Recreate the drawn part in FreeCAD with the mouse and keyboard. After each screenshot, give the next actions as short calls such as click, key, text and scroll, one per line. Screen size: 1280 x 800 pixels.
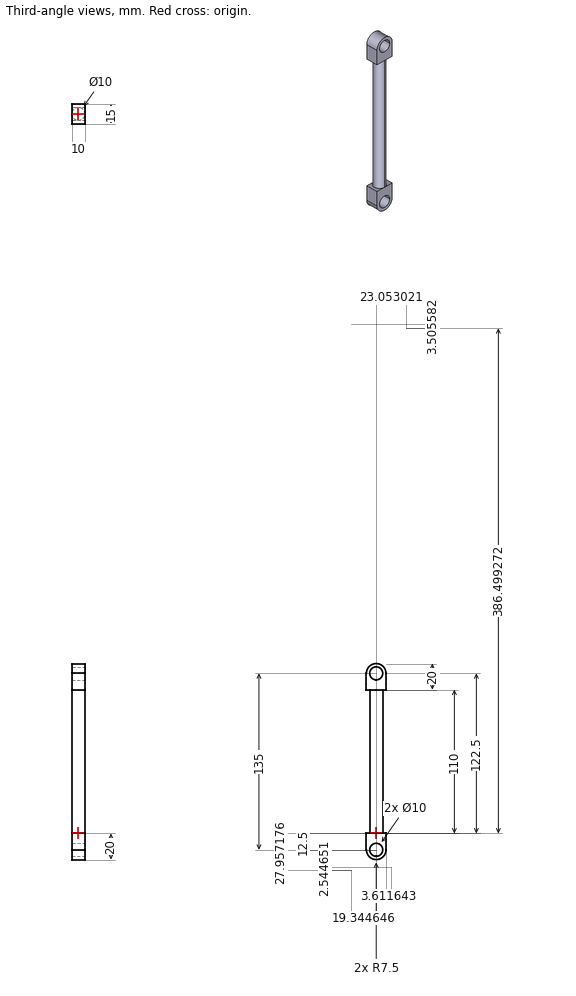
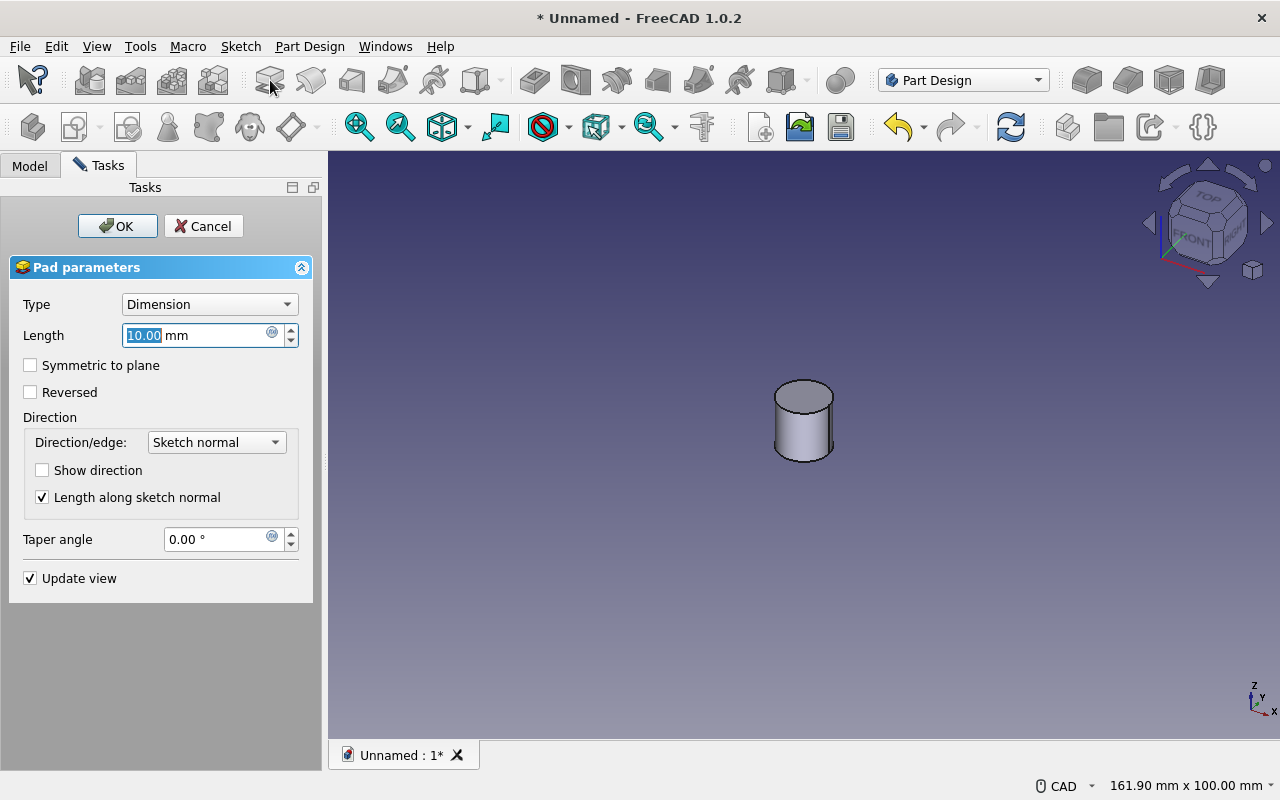
text(110)
key(Tab)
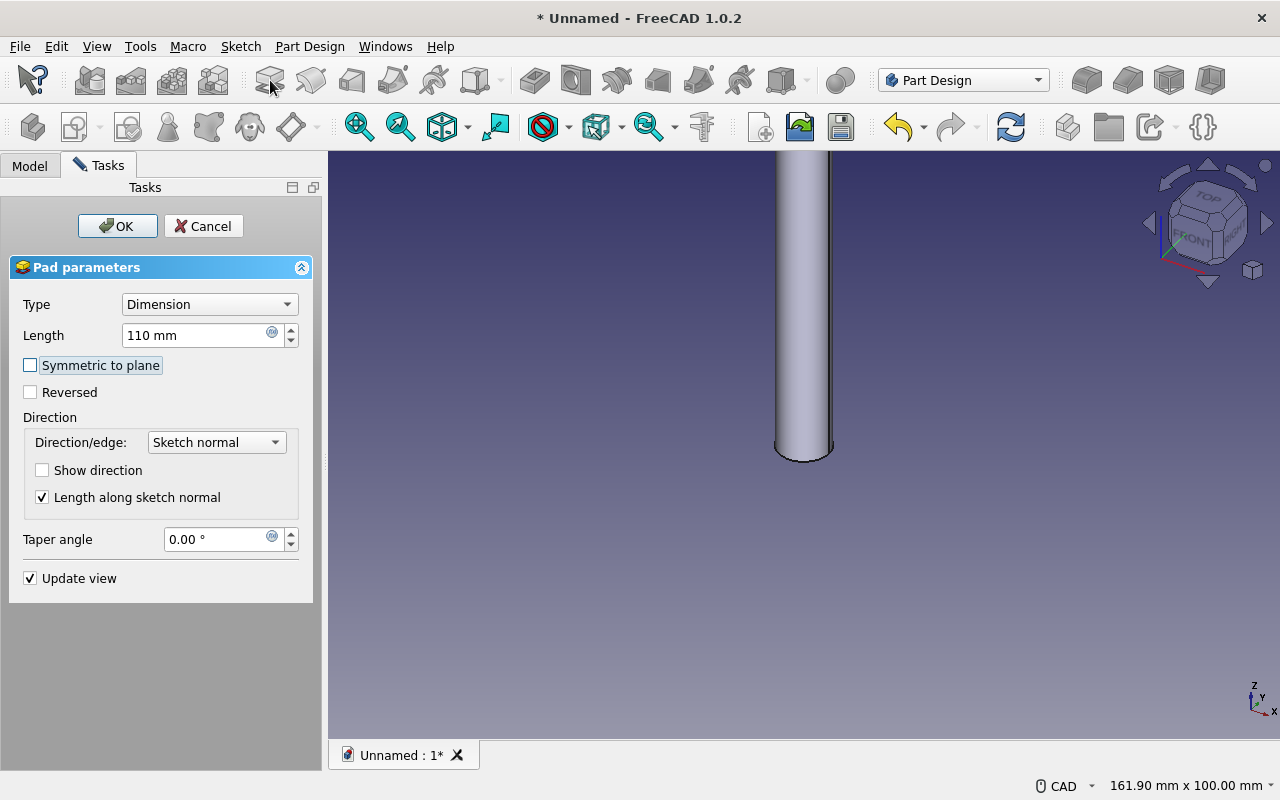
click(118, 226)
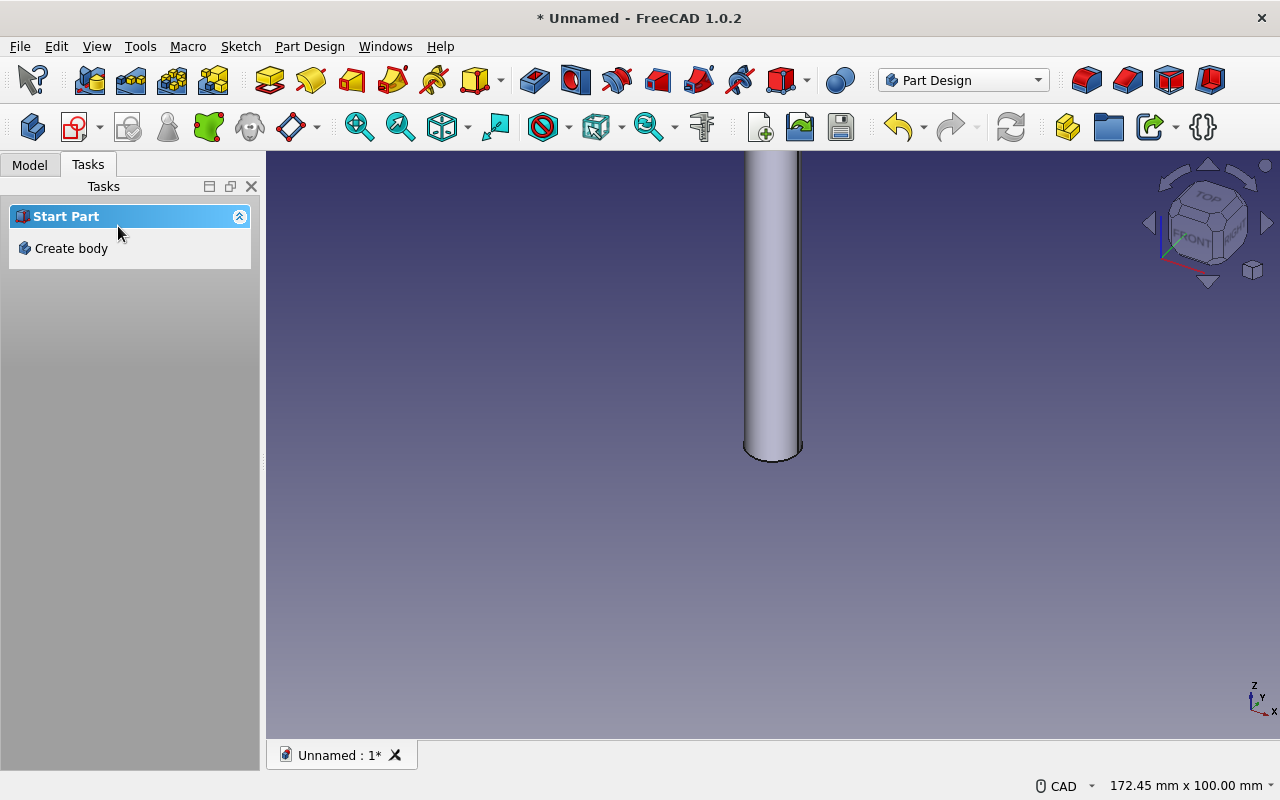
click(360, 128)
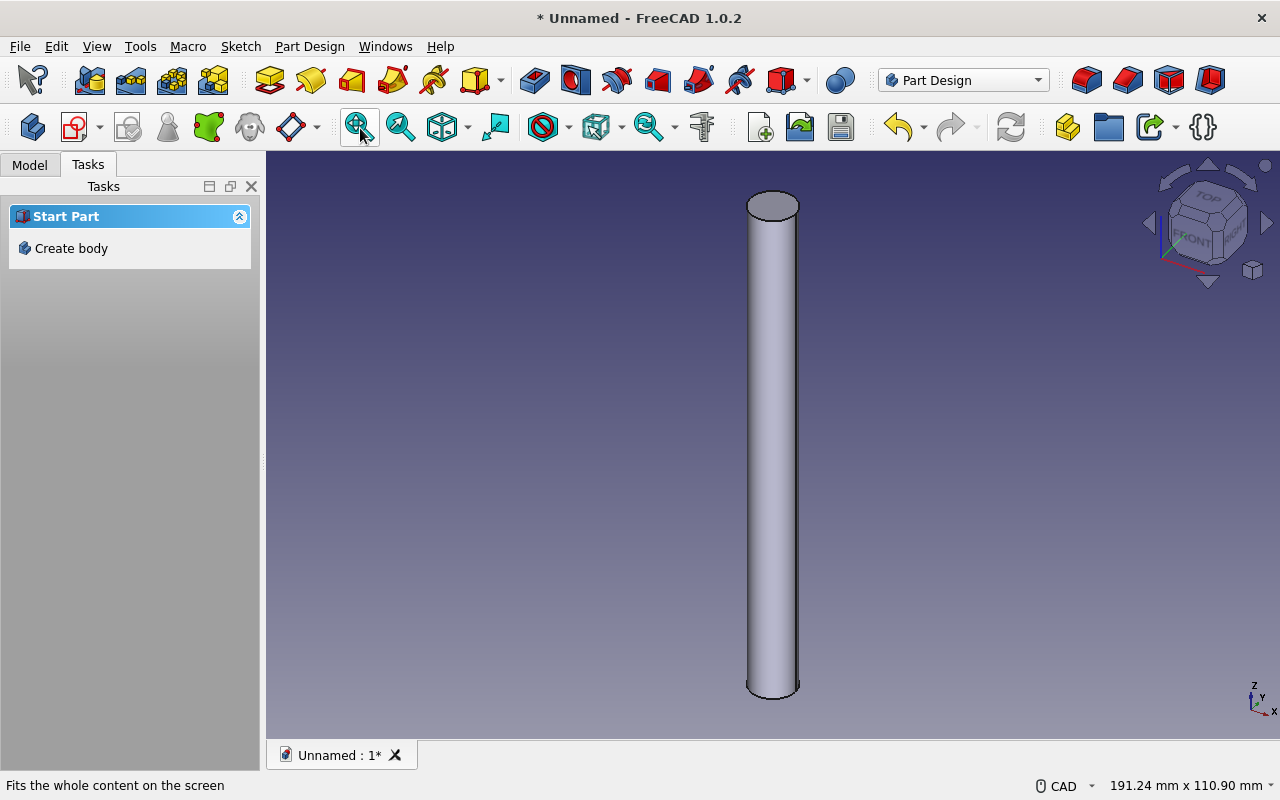
click(74, 128)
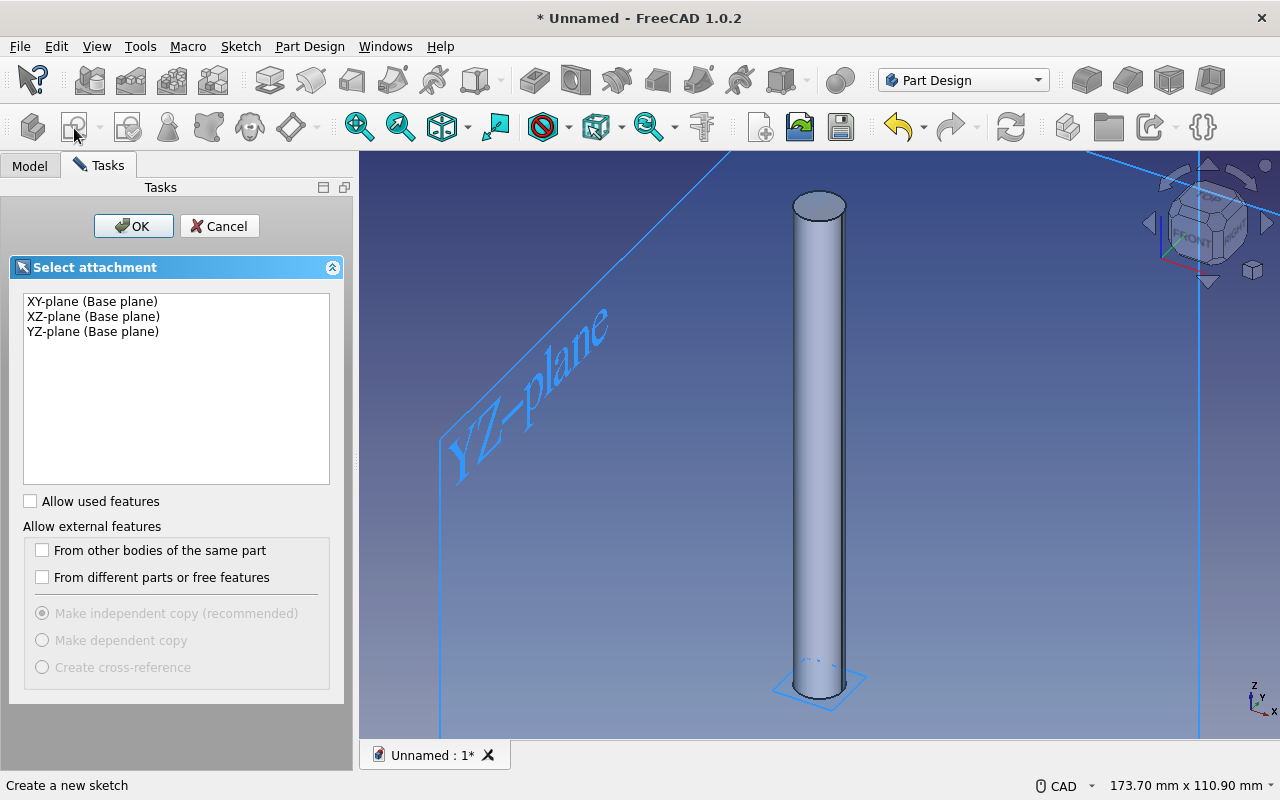
click(84, 302)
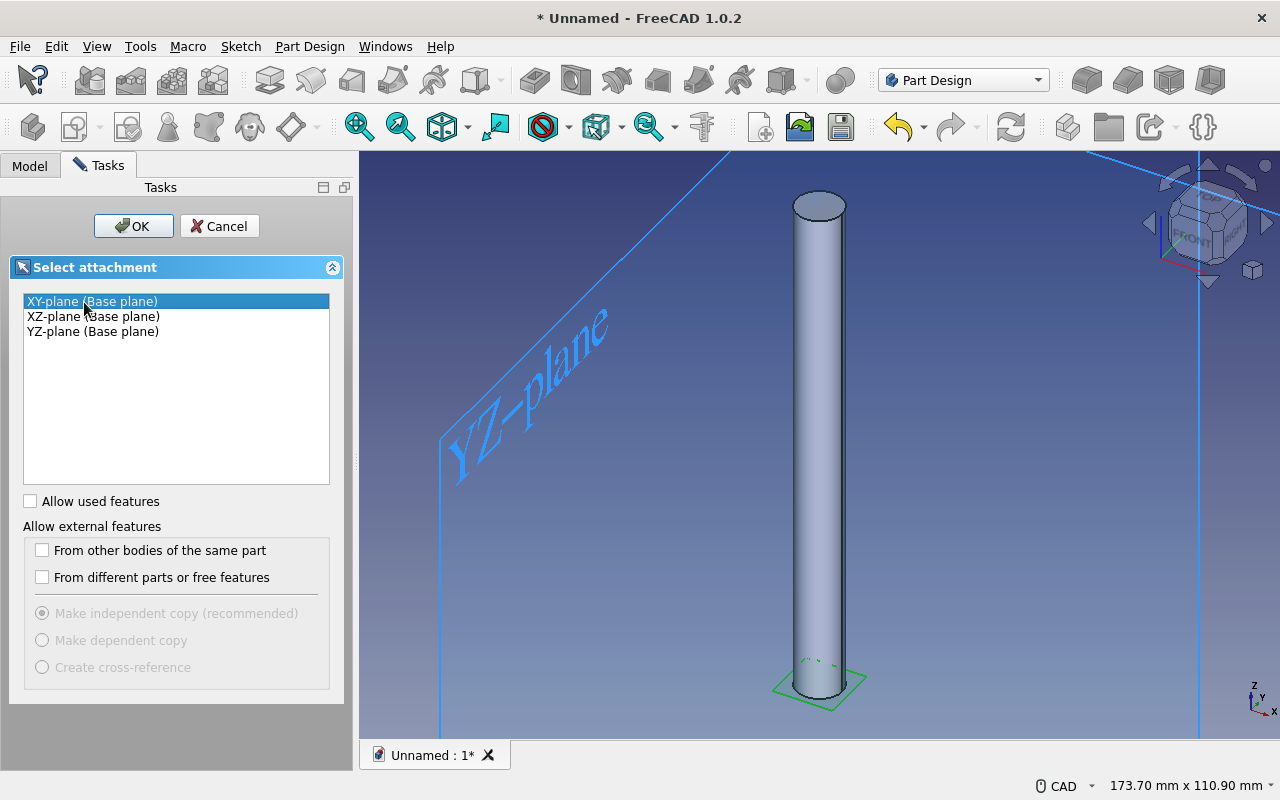
click(134, 226)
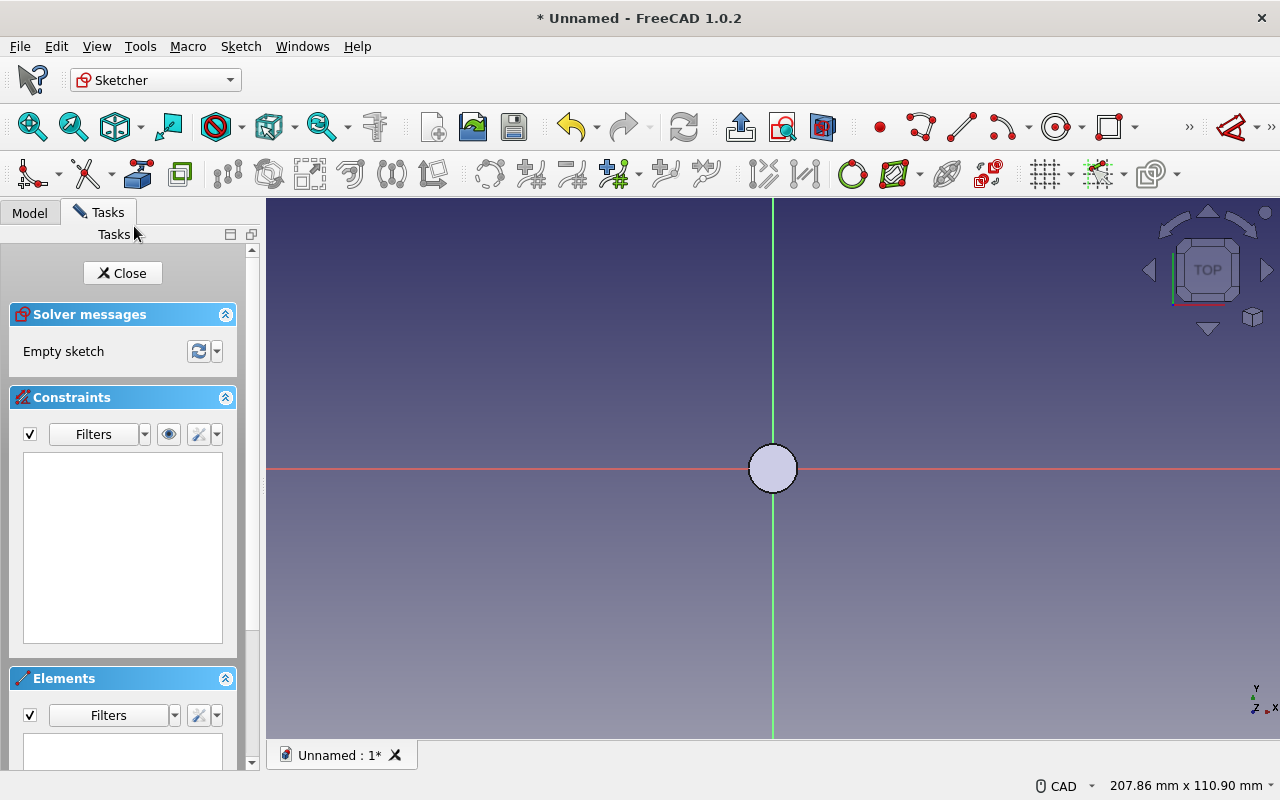
click(823, 128)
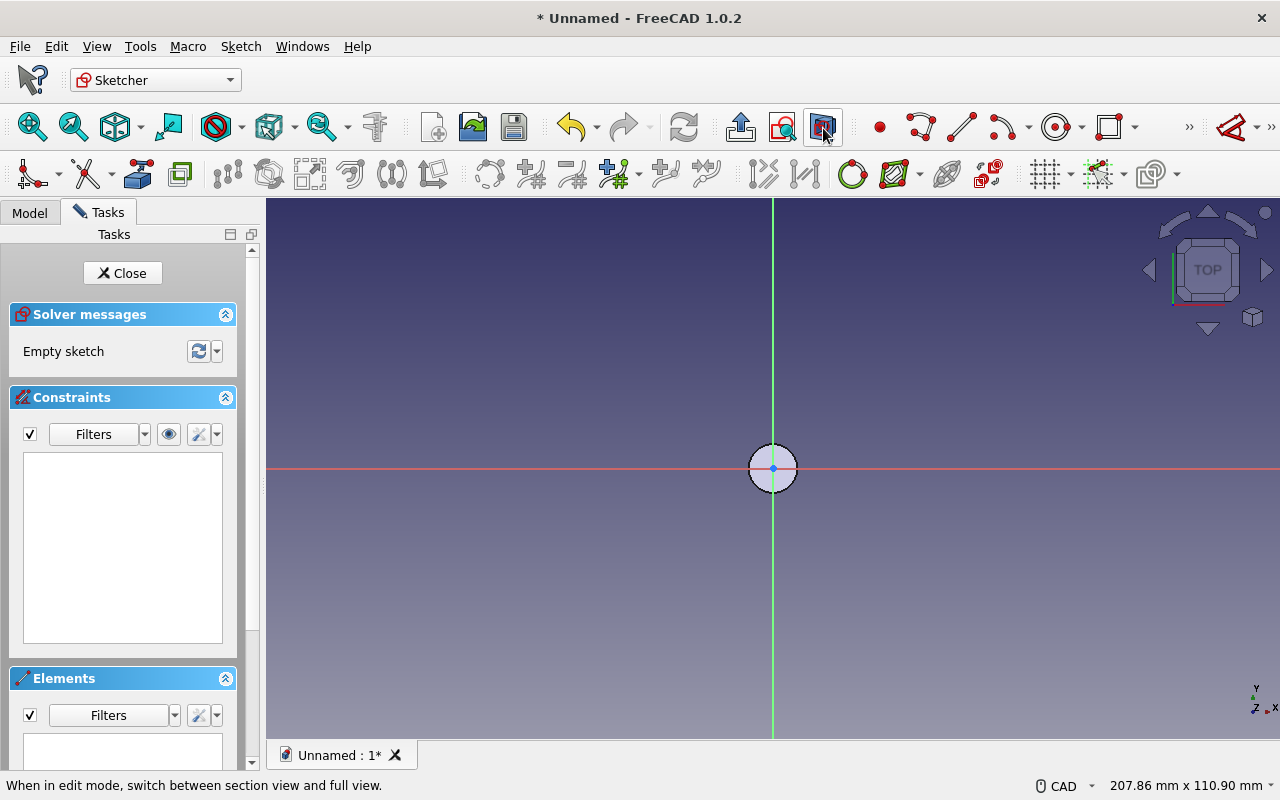
scroll(790, 469, up, 8)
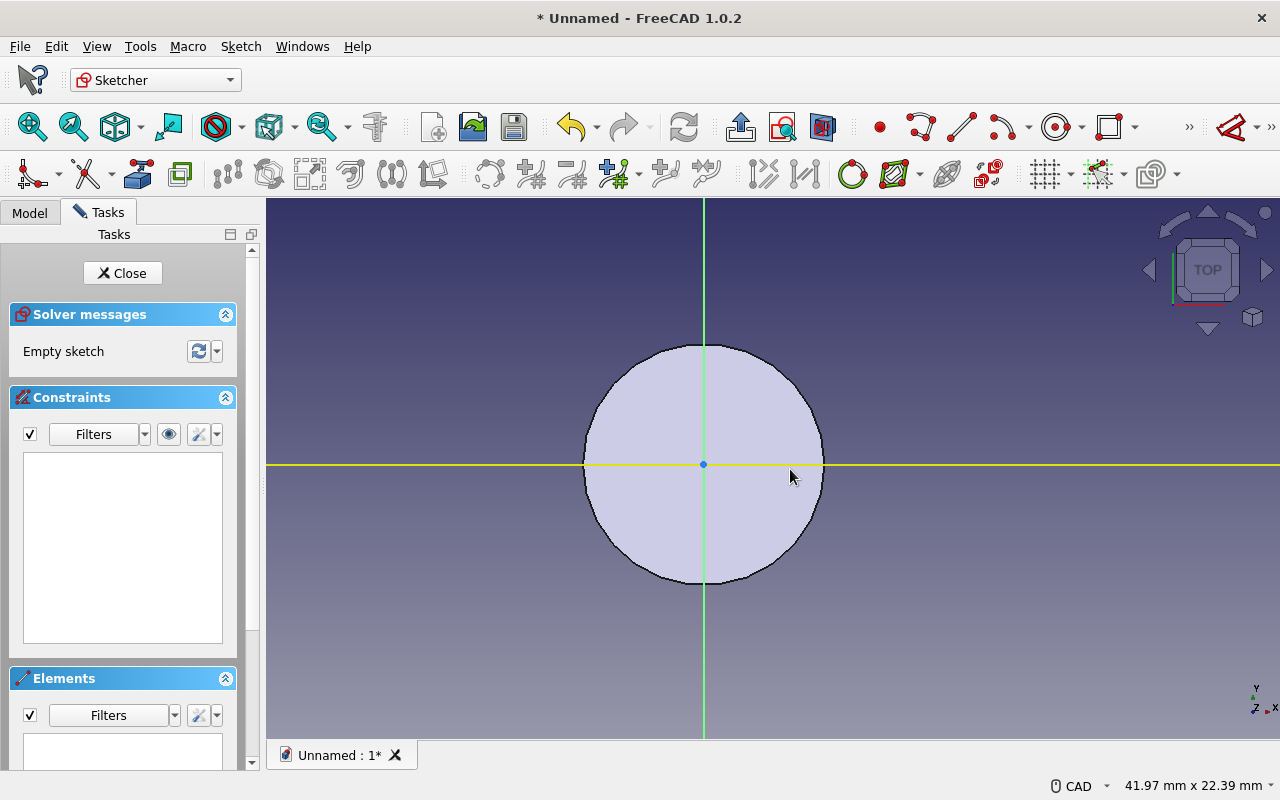
key(g)
key(v)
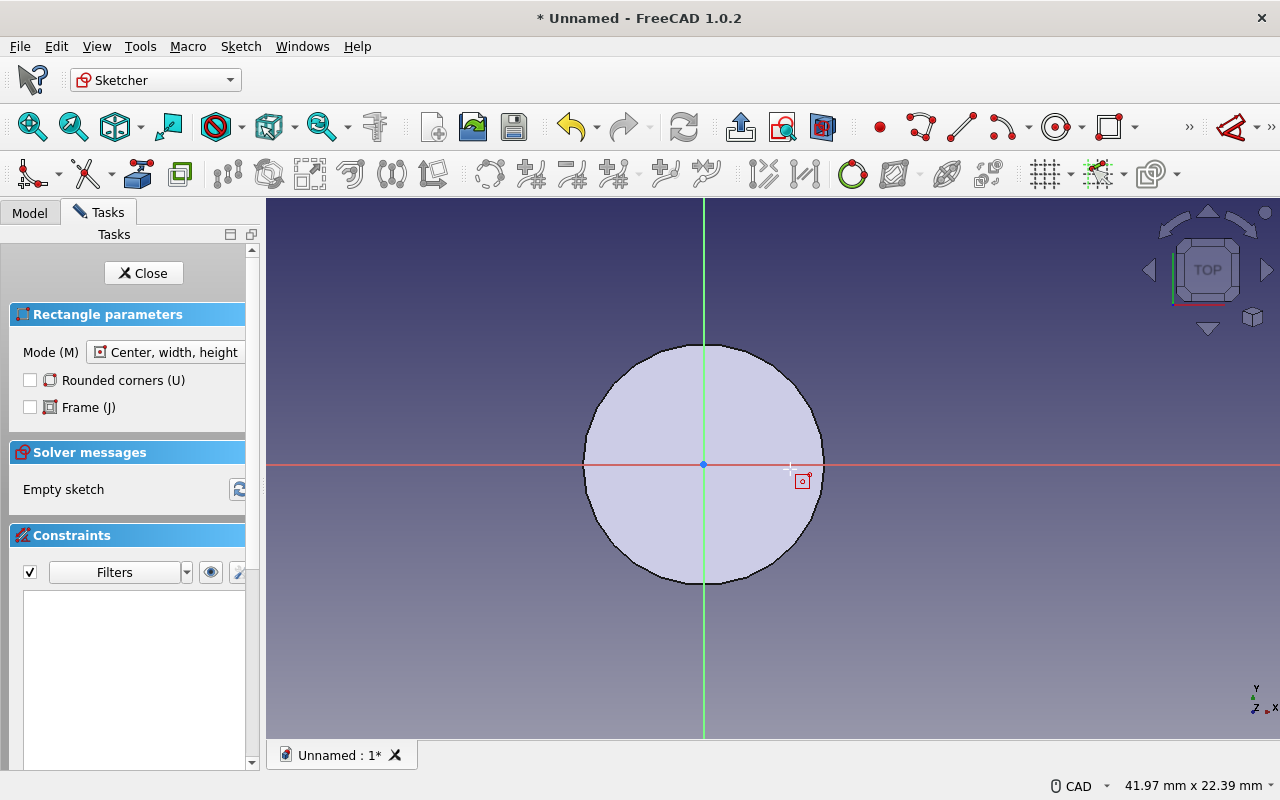
click(704, 465)
move(825, 283)